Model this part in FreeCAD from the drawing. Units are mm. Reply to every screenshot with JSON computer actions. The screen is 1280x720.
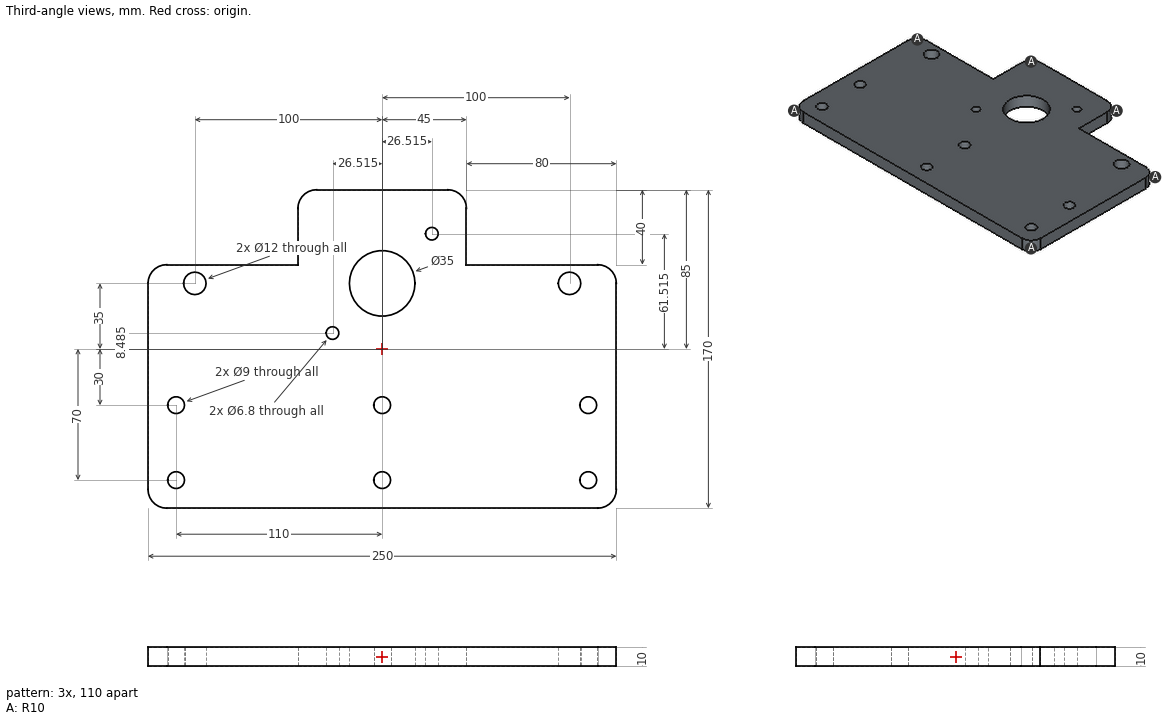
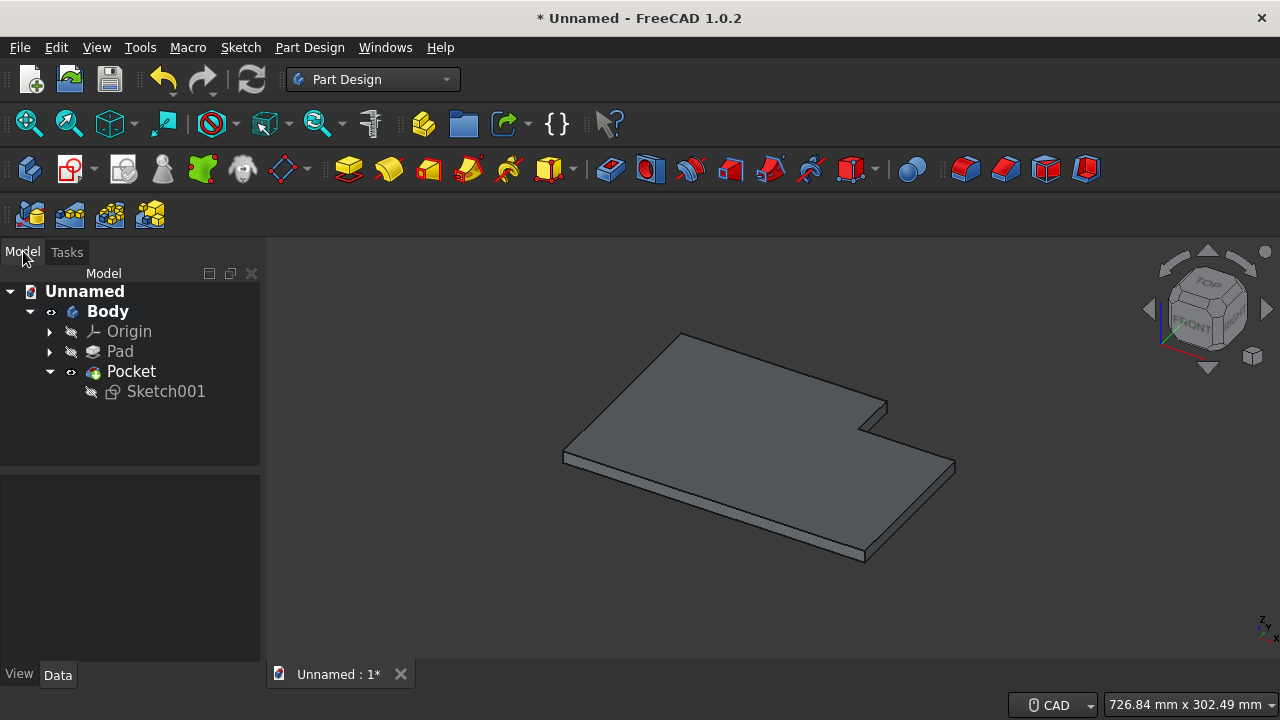
{"action": "left_click", "coordinate": [116, 372]}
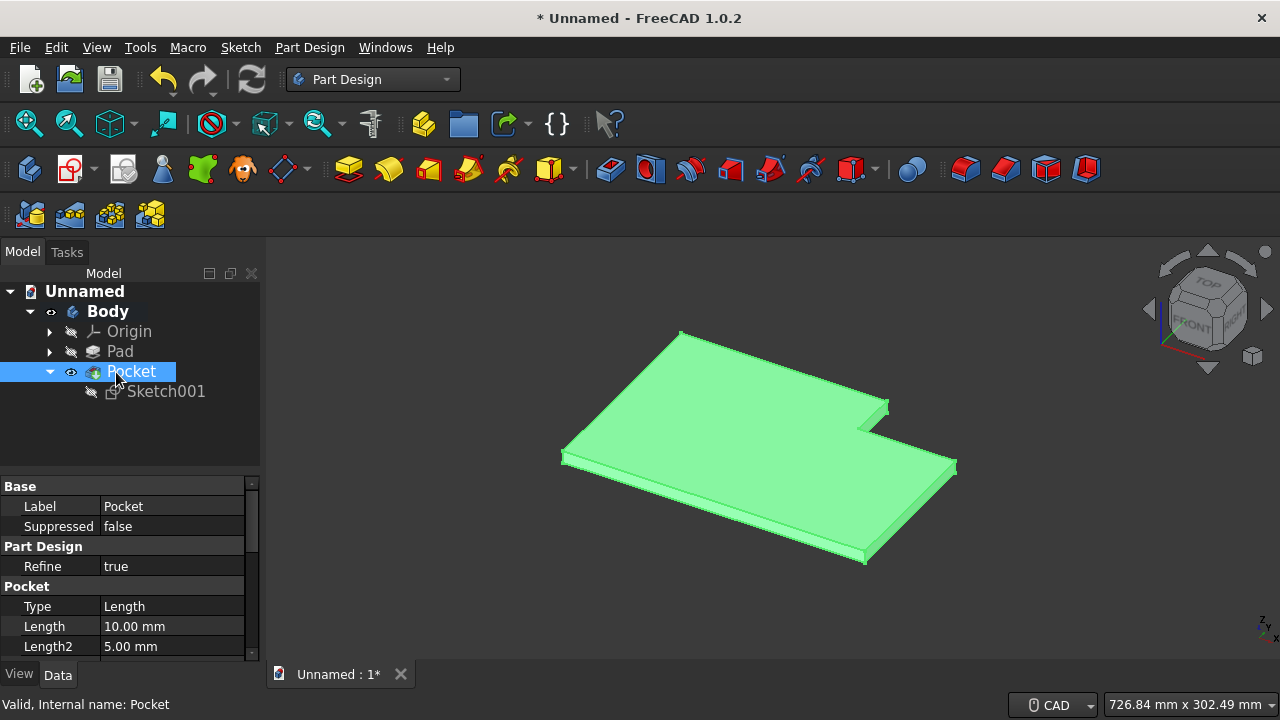
{"action": "left_click", "coordinate": [30, 214]}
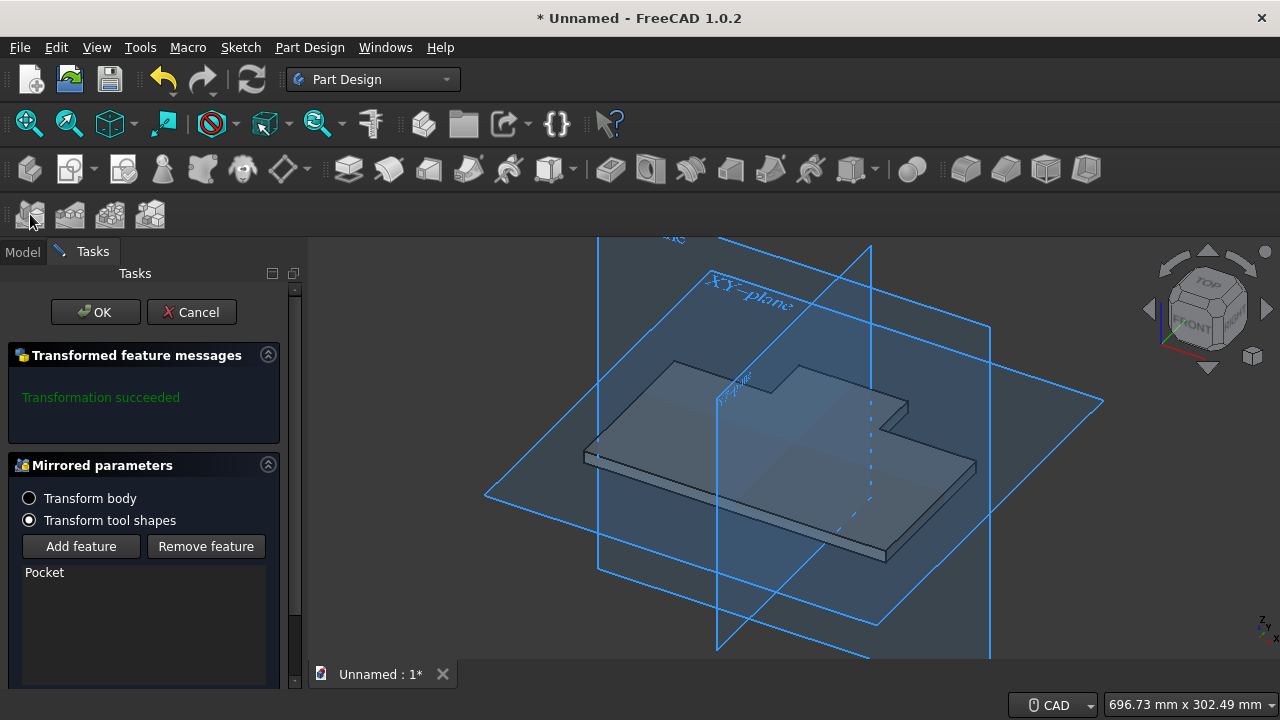
{"action": "scroll", "coordinate": [295, 486], "scroll_direction": "down", "scroll_amount": 2}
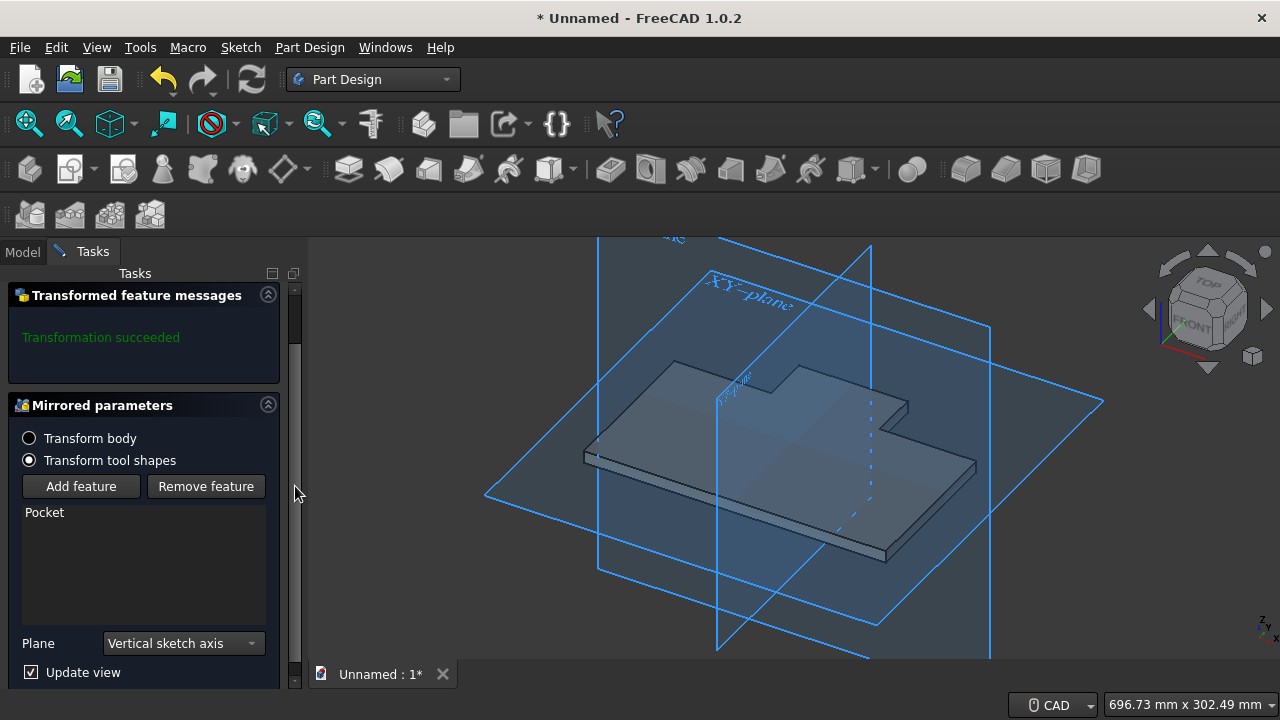
{"action": "left_click", "coordinate": [184, 628]}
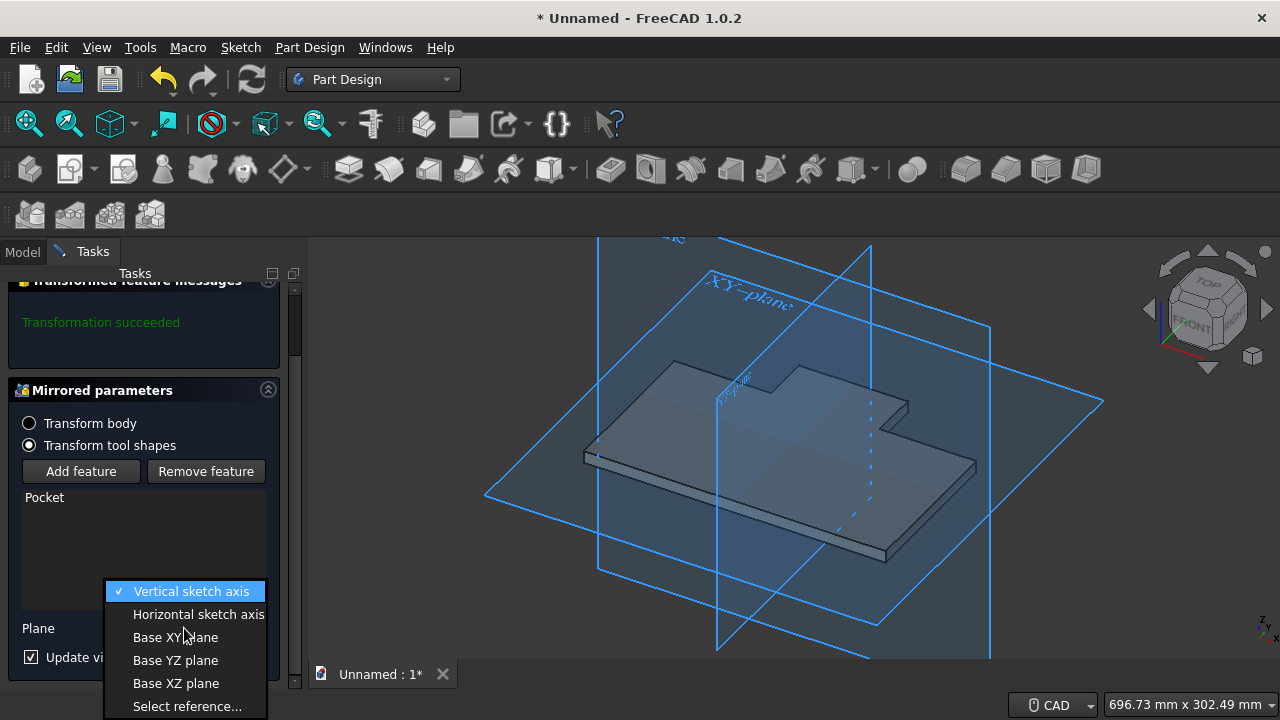
{"action": "left_click", "coordinate": [184, 660]}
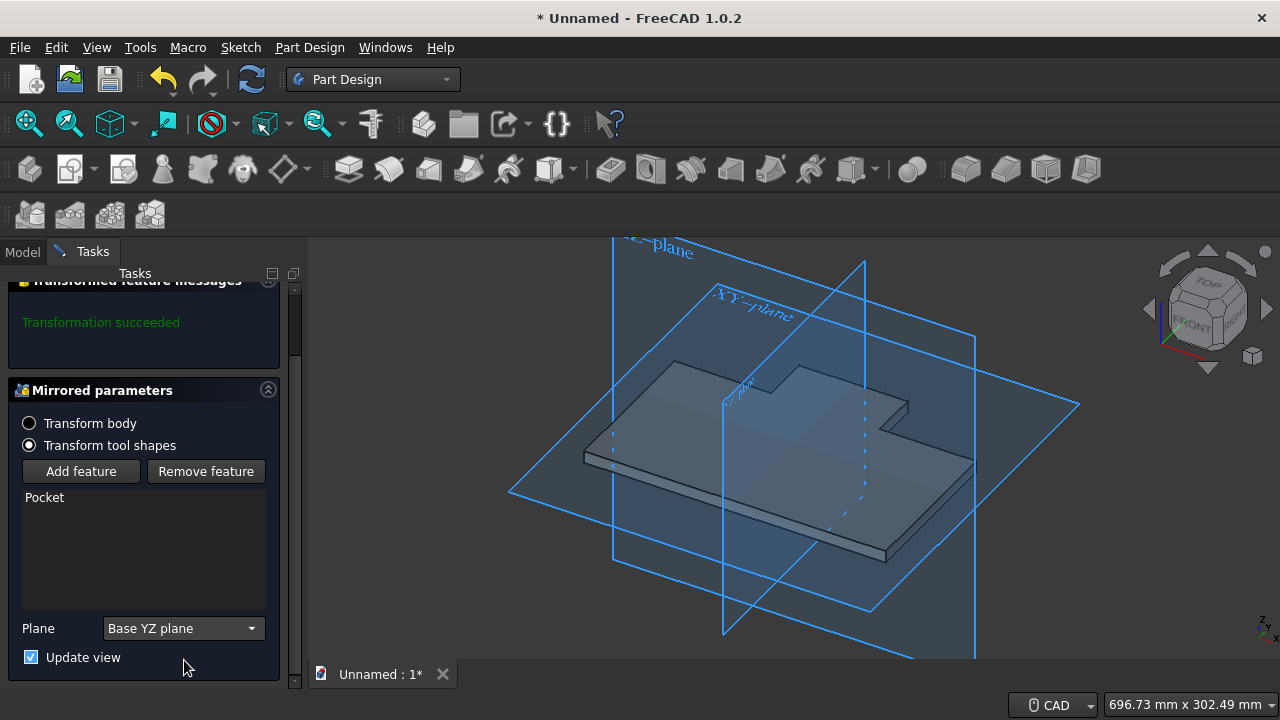
{"action": "scroll", "coordinate": [295, 486], "scroll_direction": "up", "scroll_amount": 2}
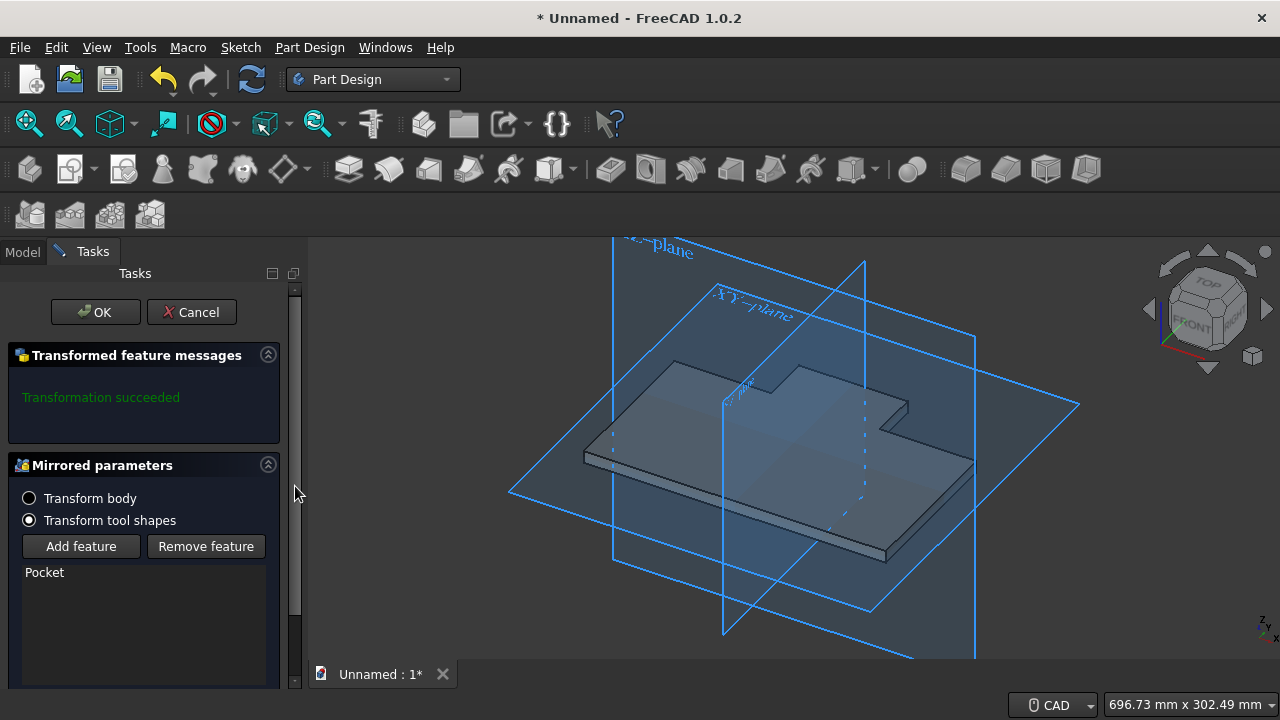
{"action": "left_click", "coordinate": [96, 312]}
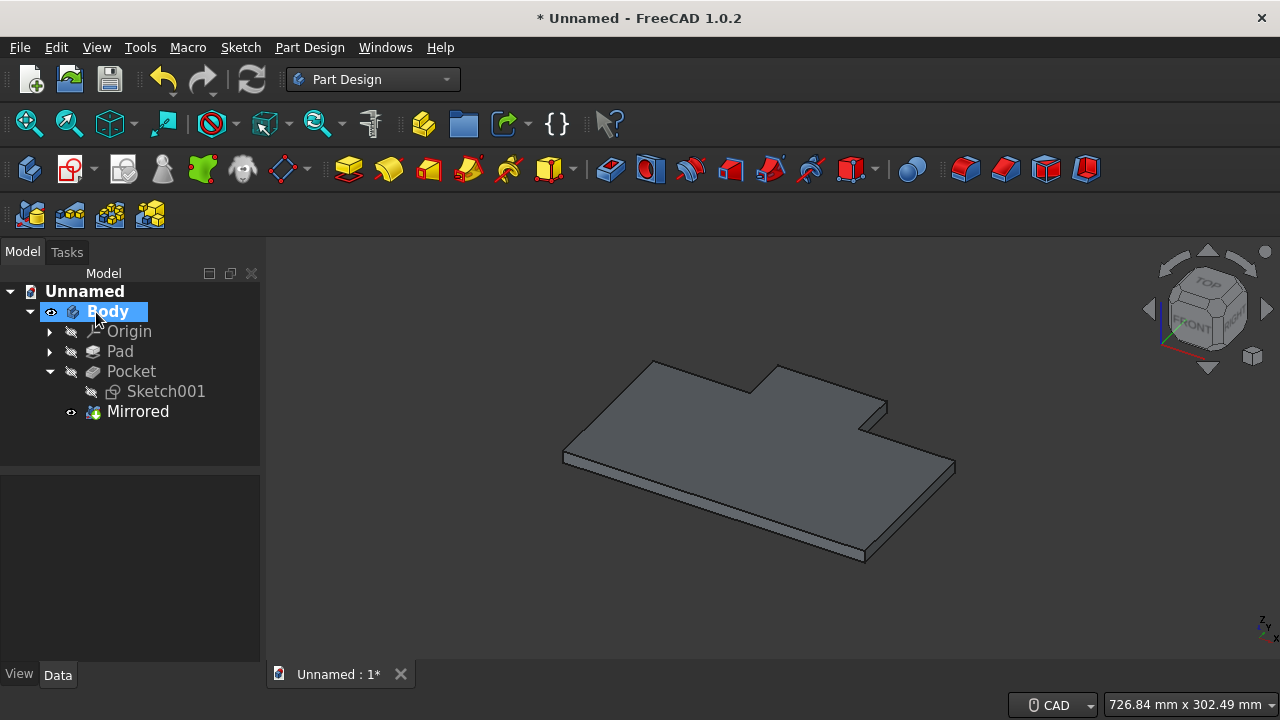
{"action": "left_click", "coordinate": [773, 441]}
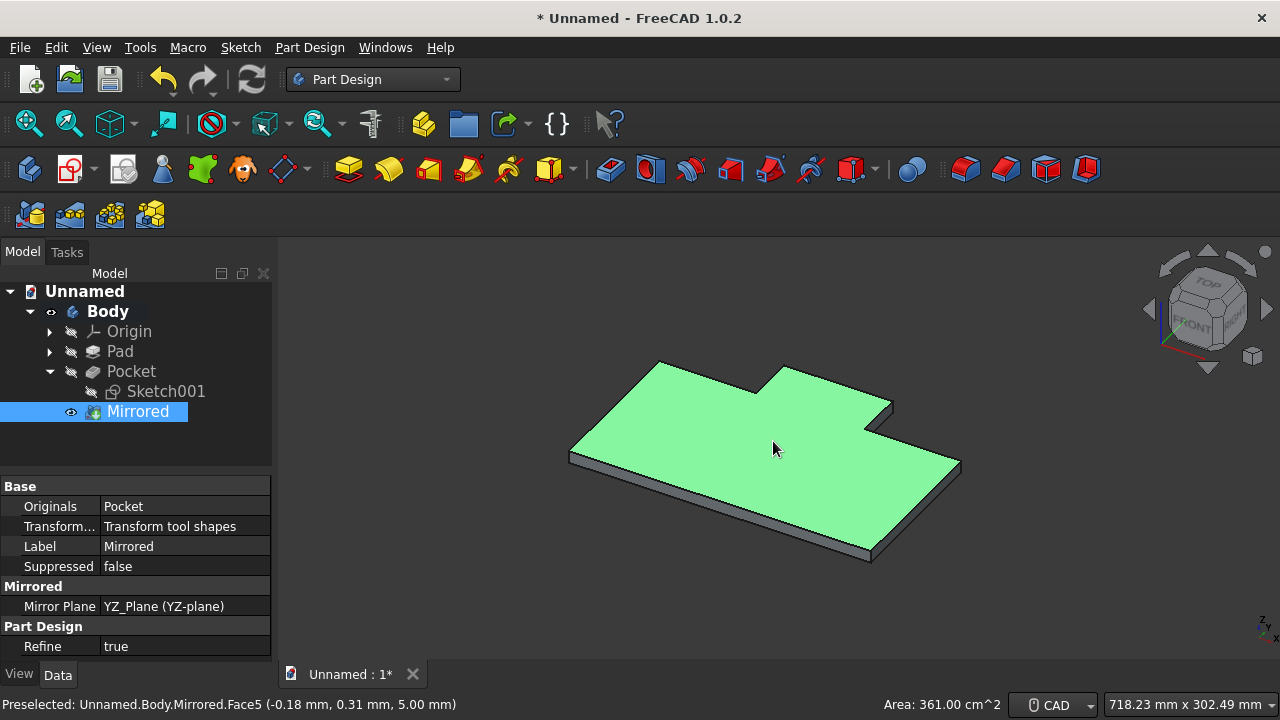
{"action": "left_click", "coordinate": [70, 170]}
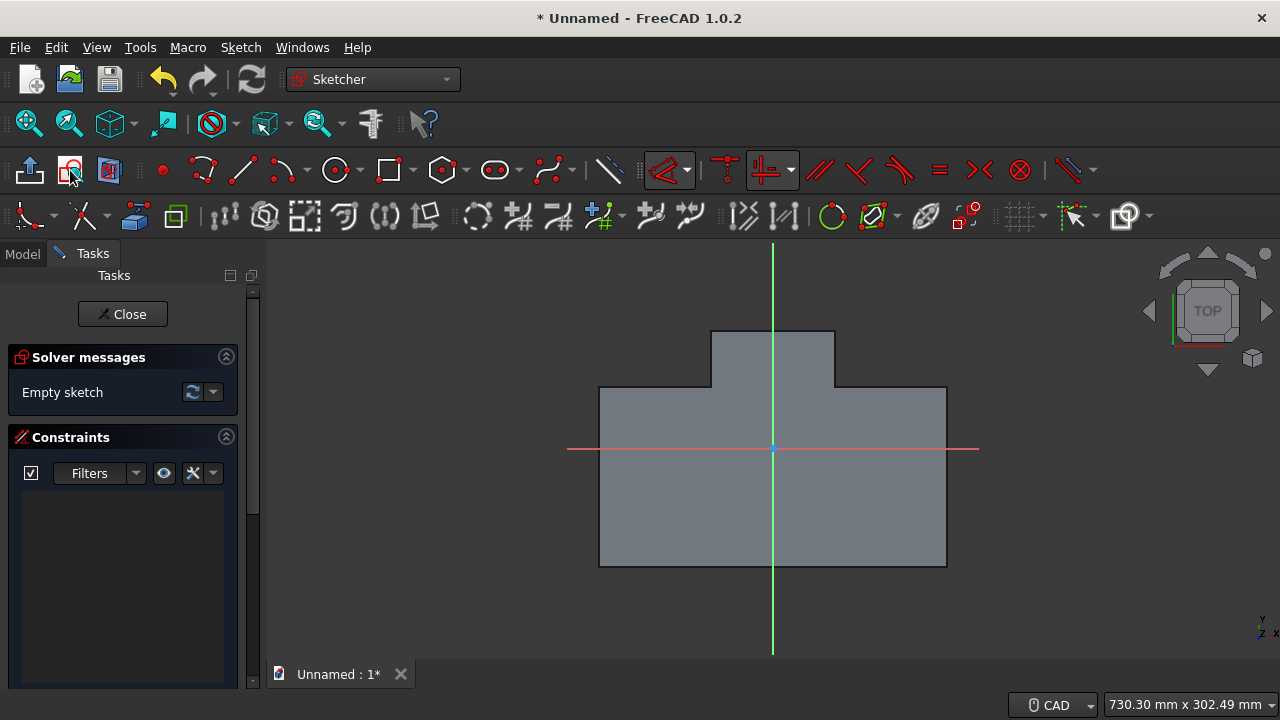
{"action": "scroll", "coordinate": [687, 531], "scroll_direction": "up", "scroll_amount": 5}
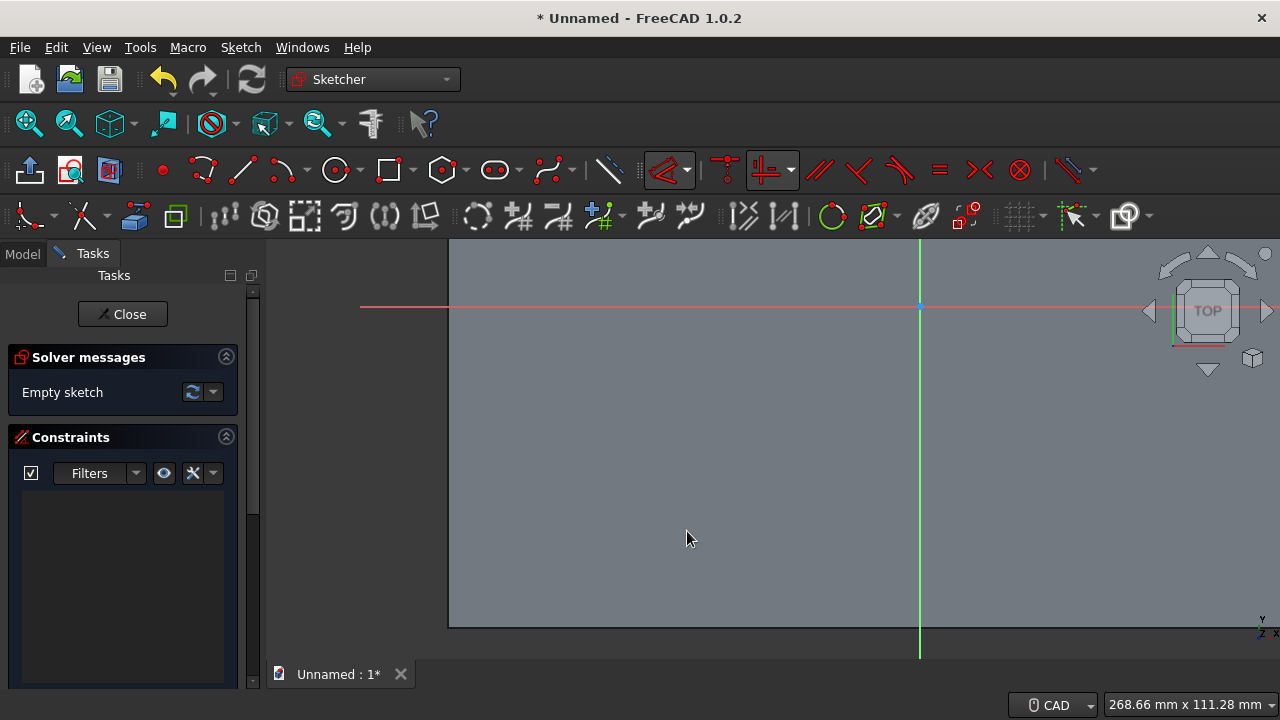
{"action": "left_click", "coordinate": [336, 170]}